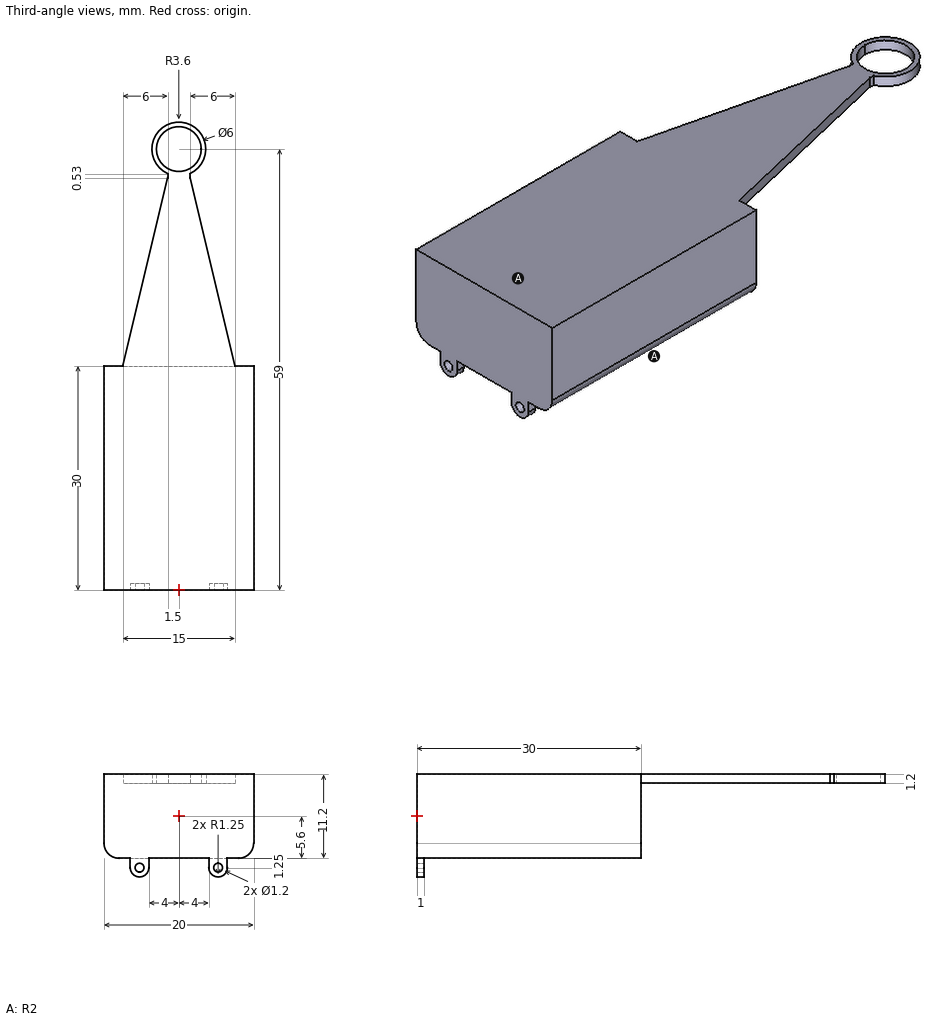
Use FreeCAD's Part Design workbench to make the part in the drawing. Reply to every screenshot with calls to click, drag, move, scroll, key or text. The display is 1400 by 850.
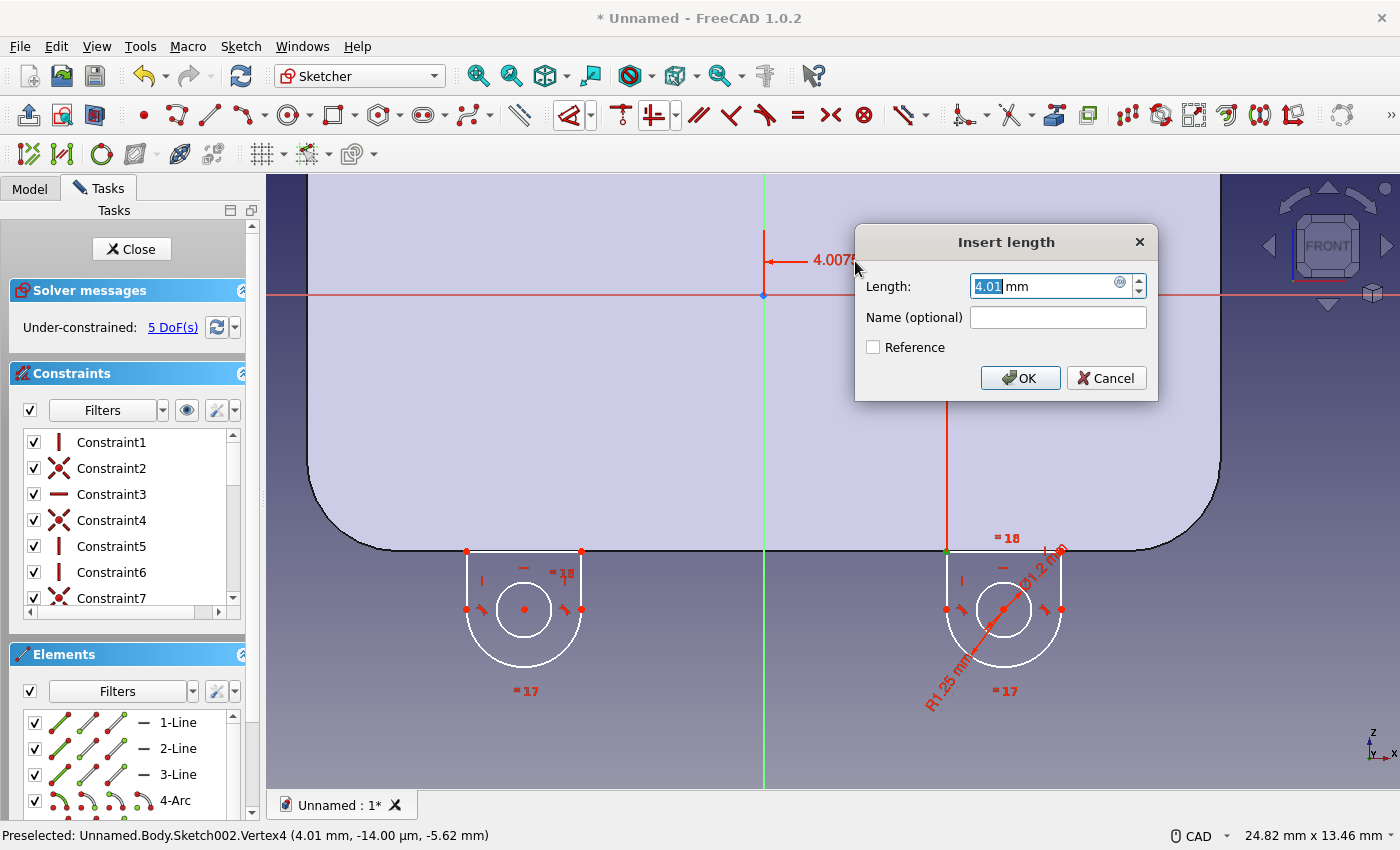
text(4)
key(Return)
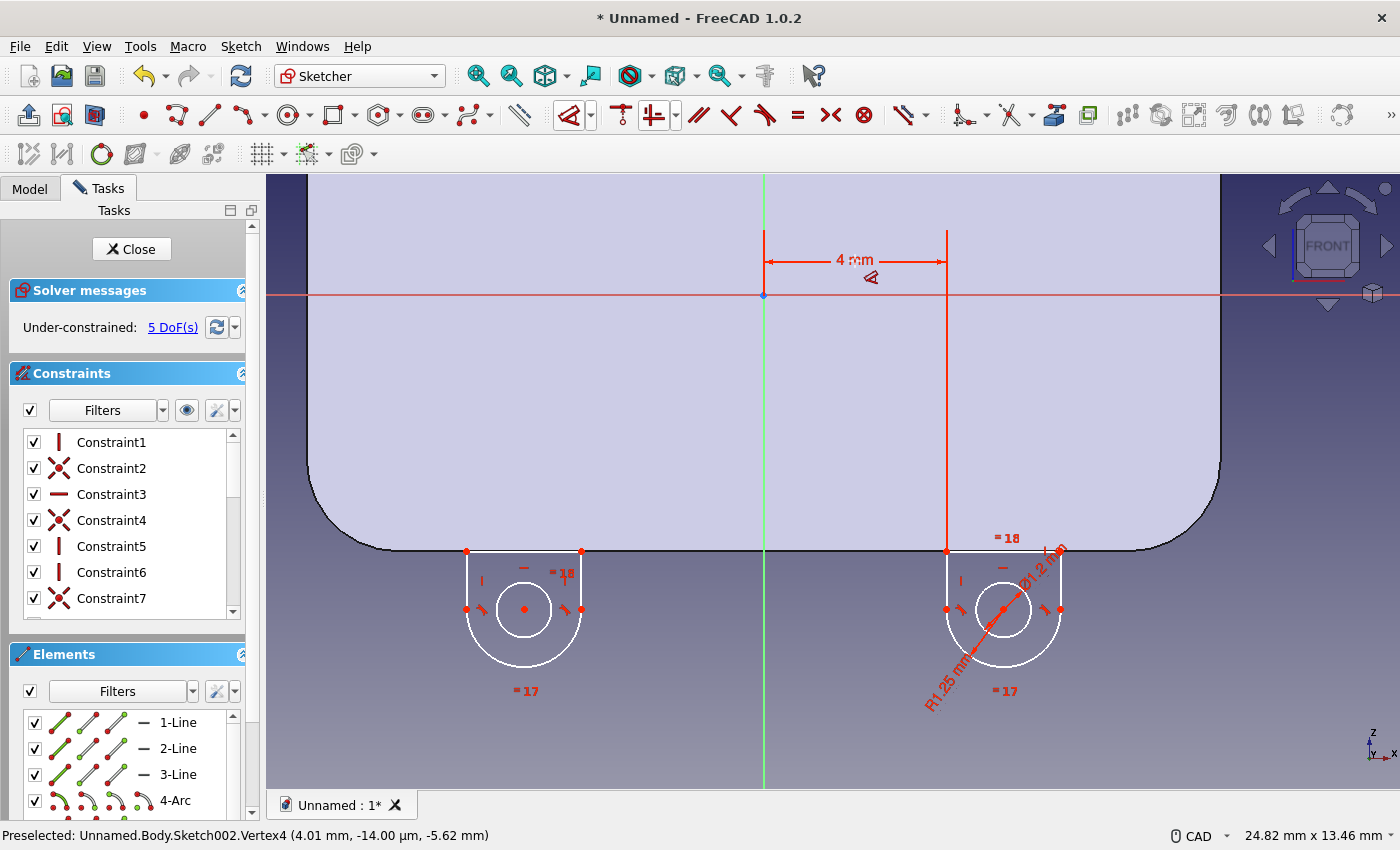
click(581, 610)
click(672, 261)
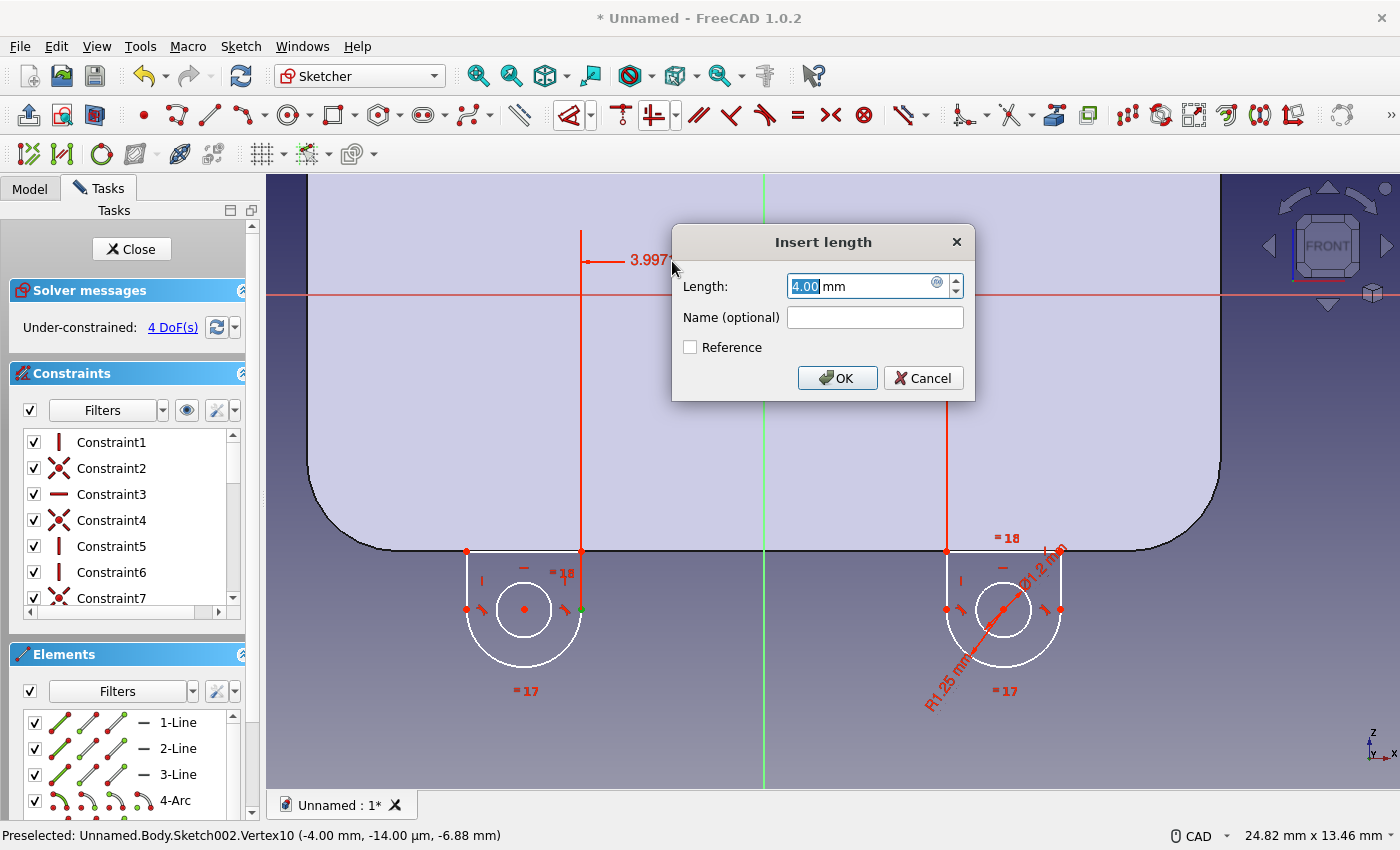
text(4)
key(Return)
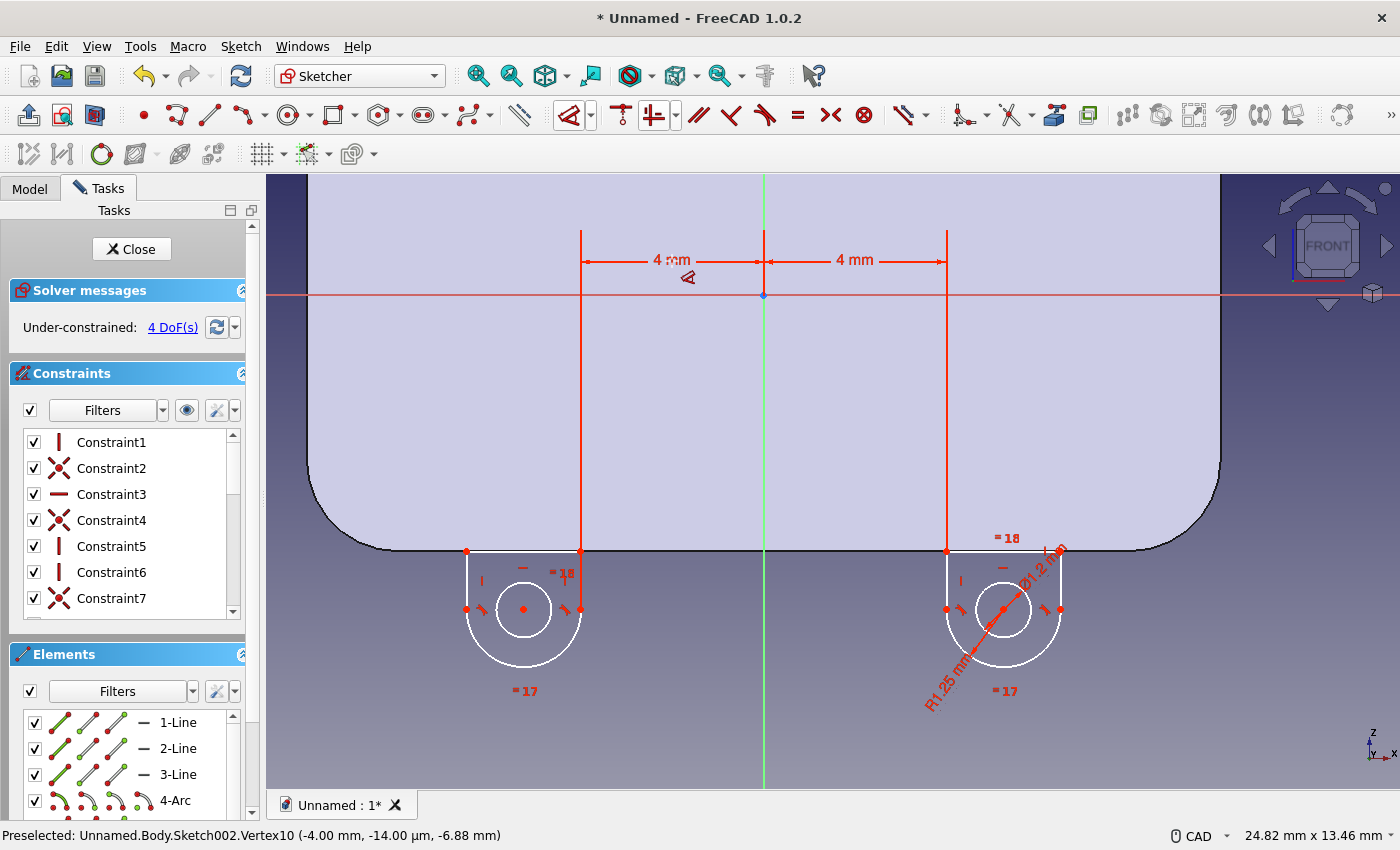
click(1061, 593)
click(1095, 594)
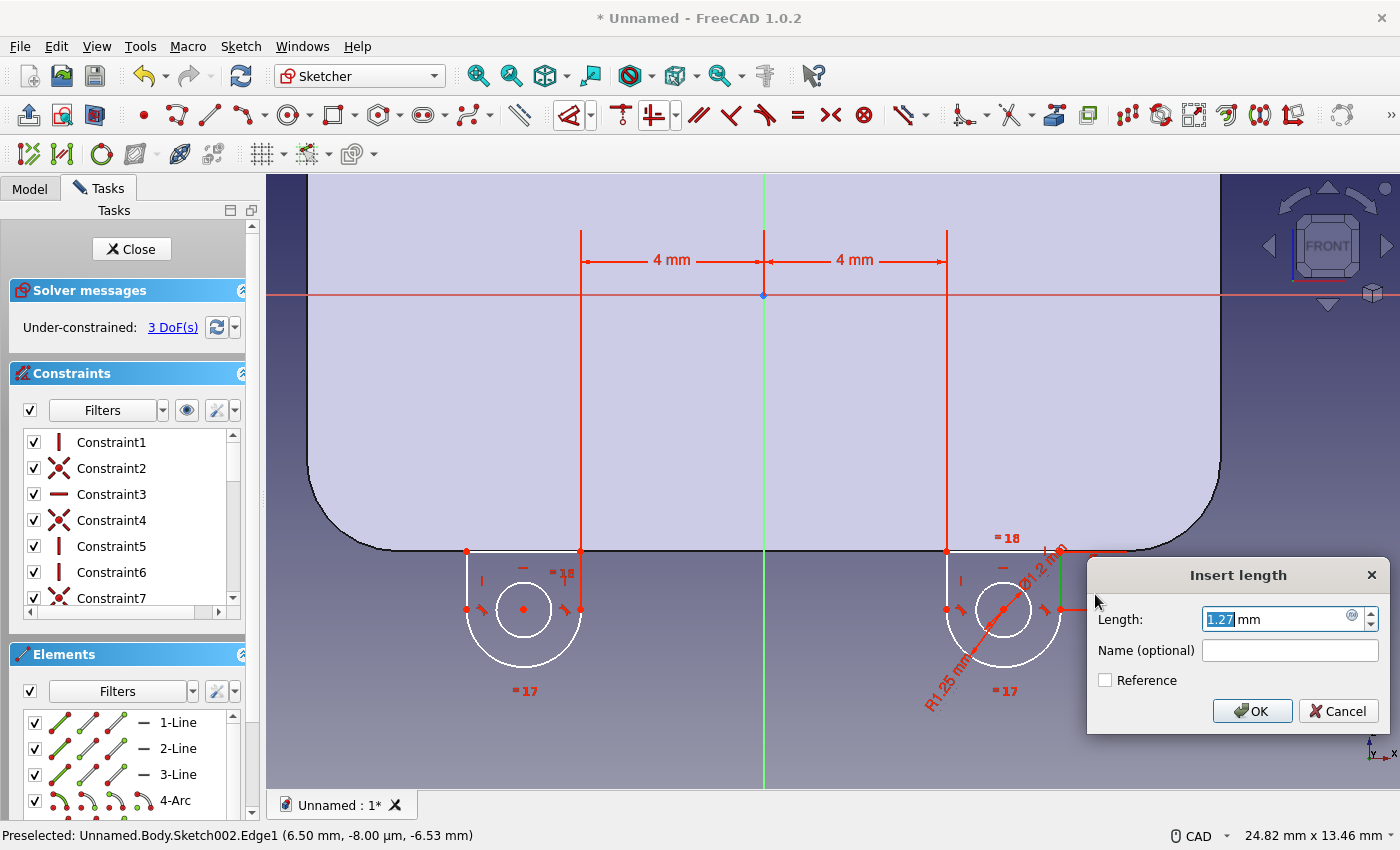
text(1.25)
key(Return)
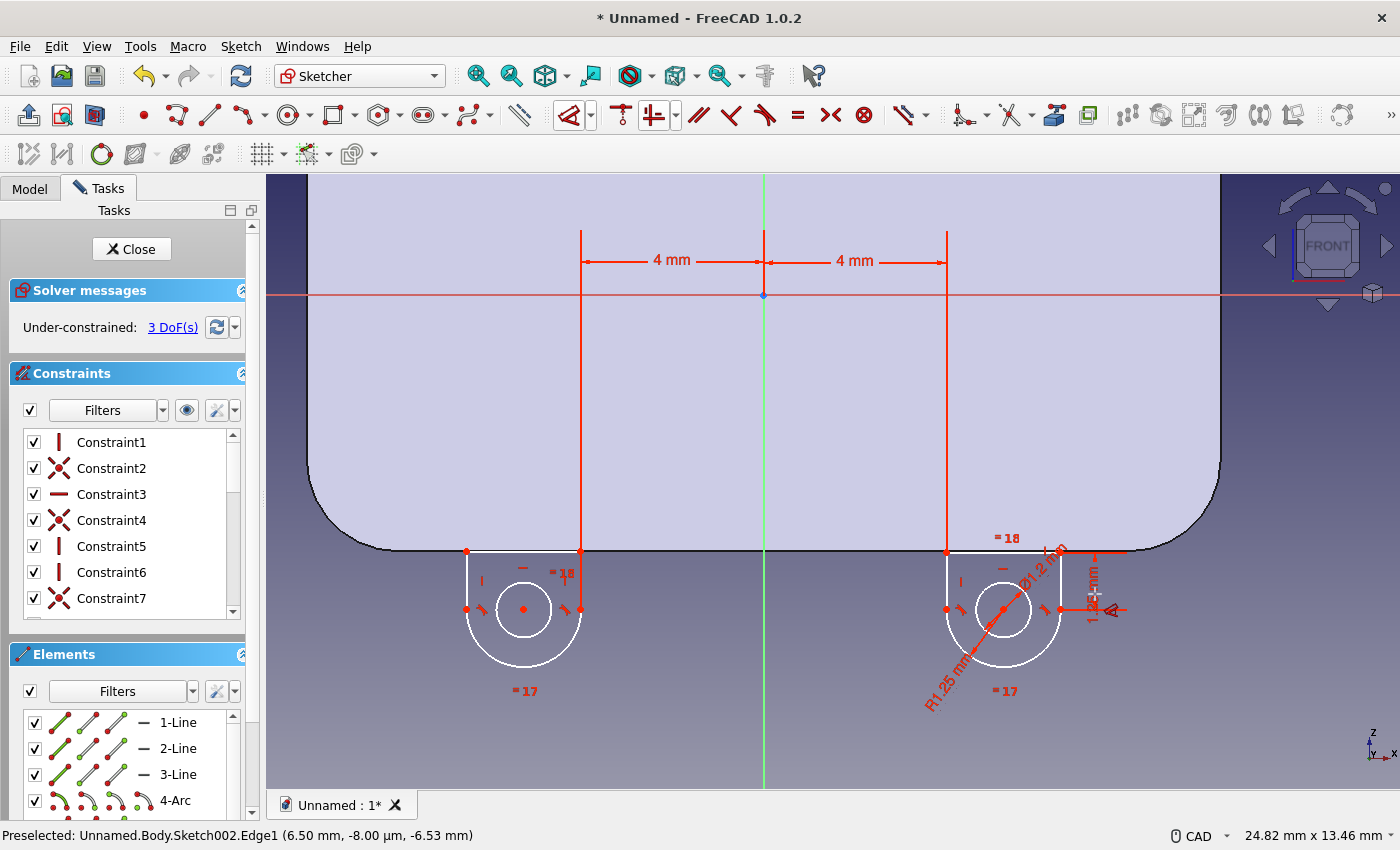
click(581, 593)
click(547, 568)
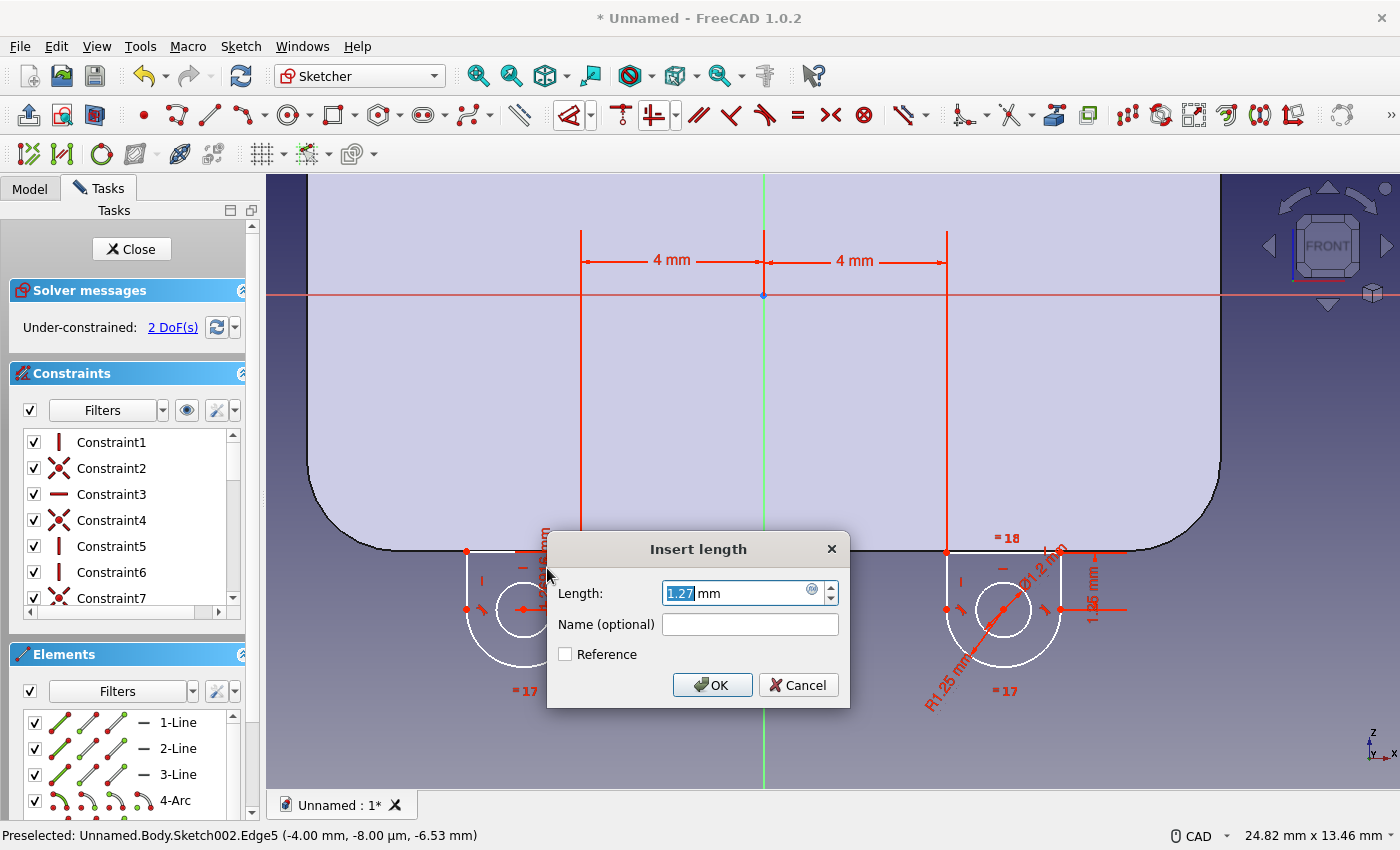
text(1.25)
key(Return)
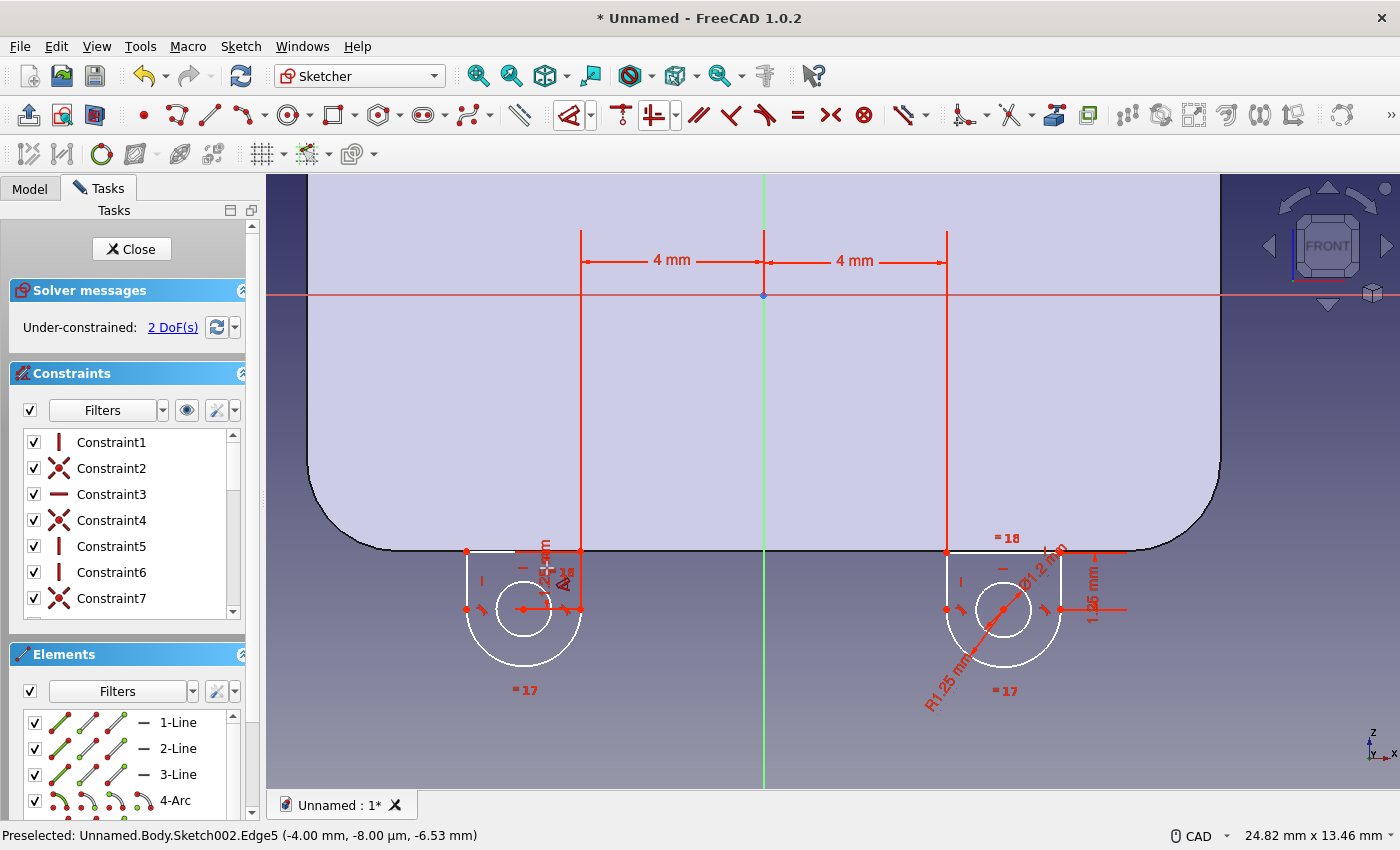
click(1061, 553)
click(1095, 424)